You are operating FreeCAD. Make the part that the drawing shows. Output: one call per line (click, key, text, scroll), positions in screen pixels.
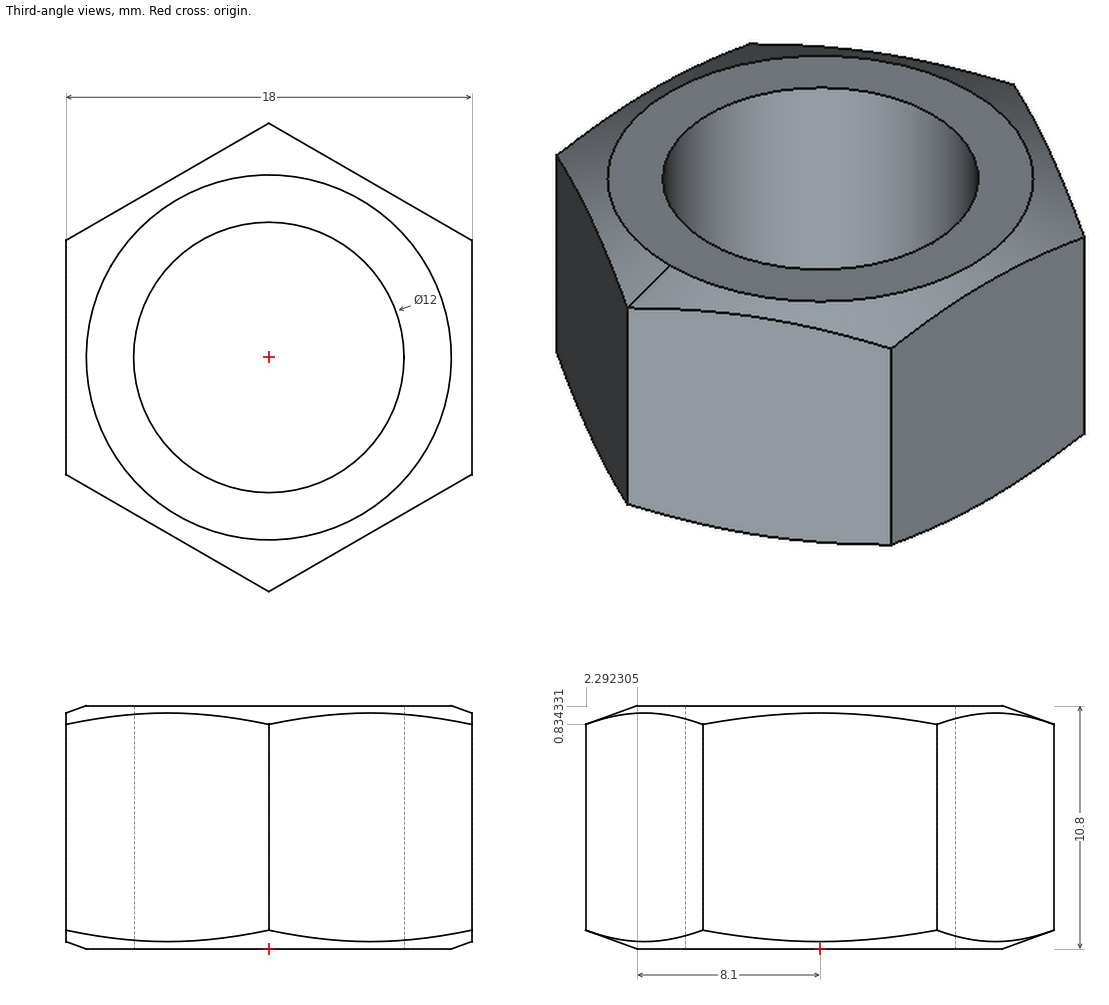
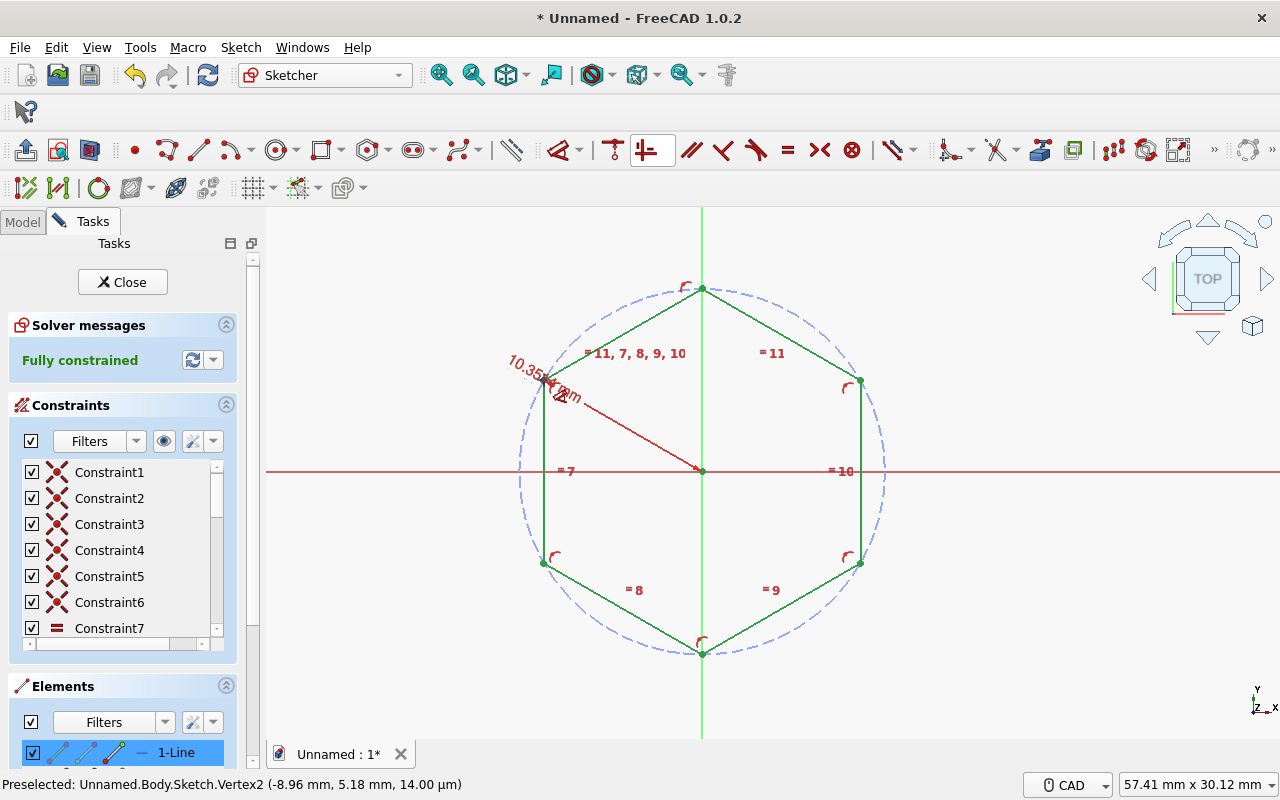
click(861, 563)
click(629, 597)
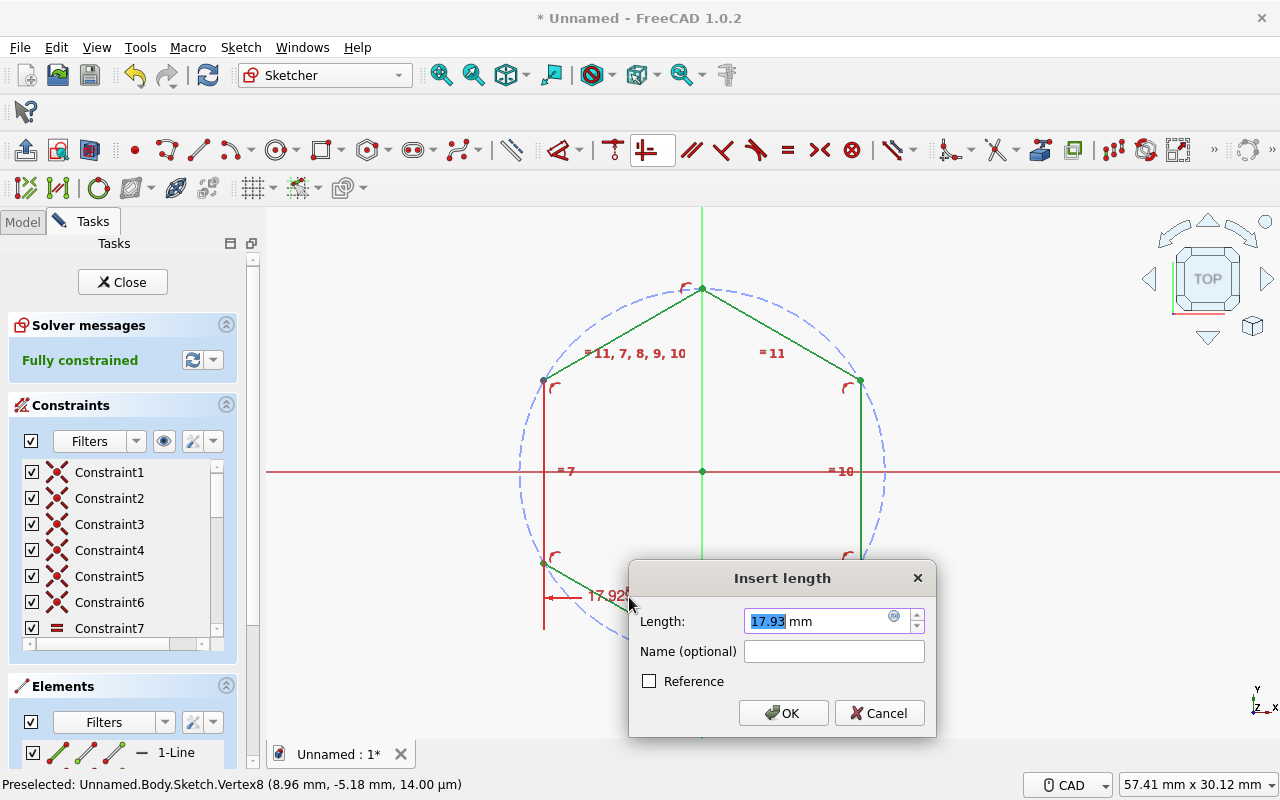
text(18)
key(Return)
key(Escape)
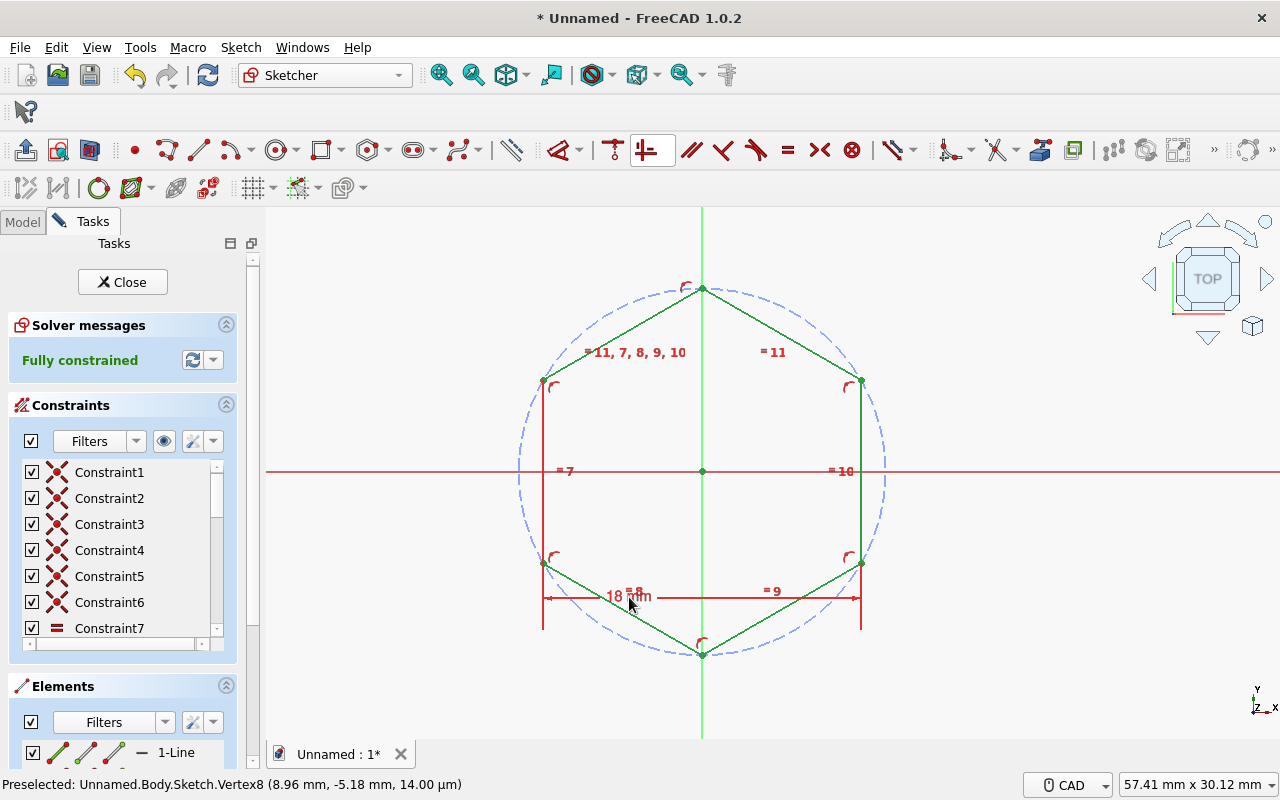
click(123, 282)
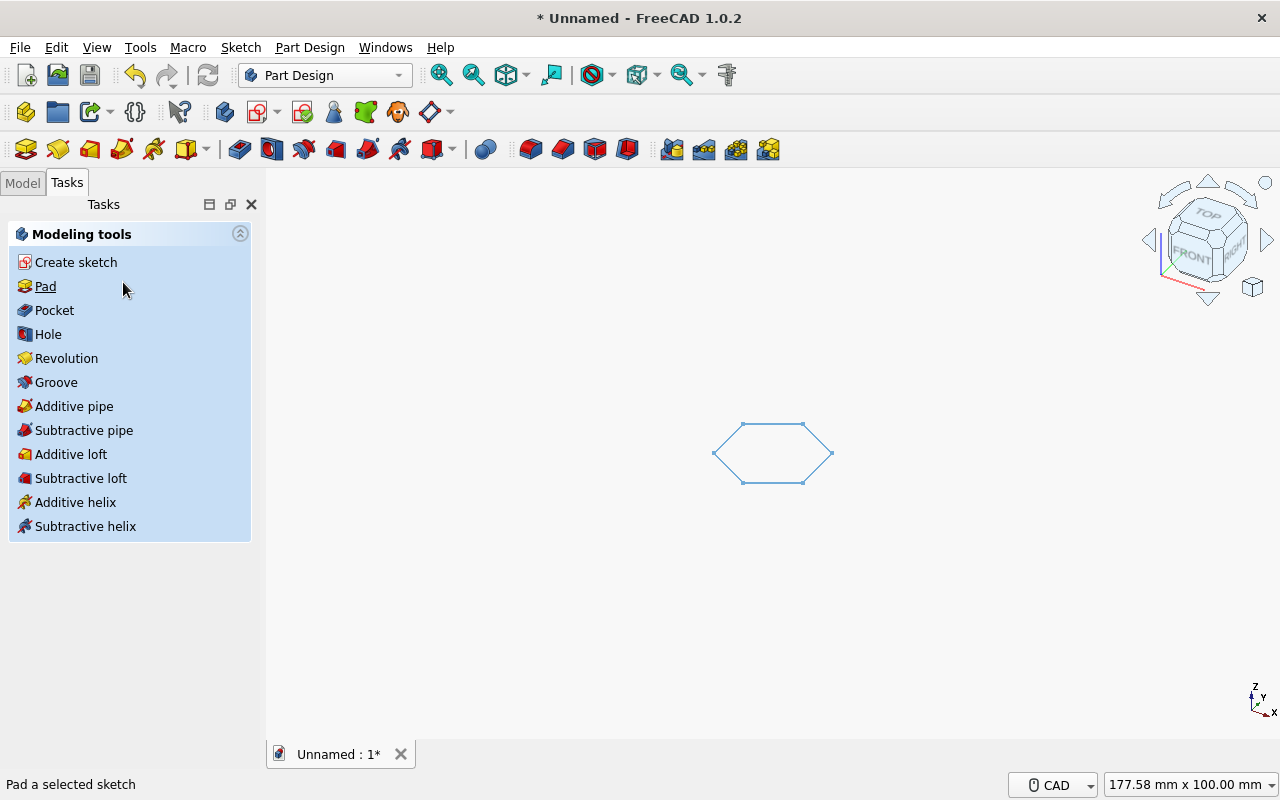
click(26, 150)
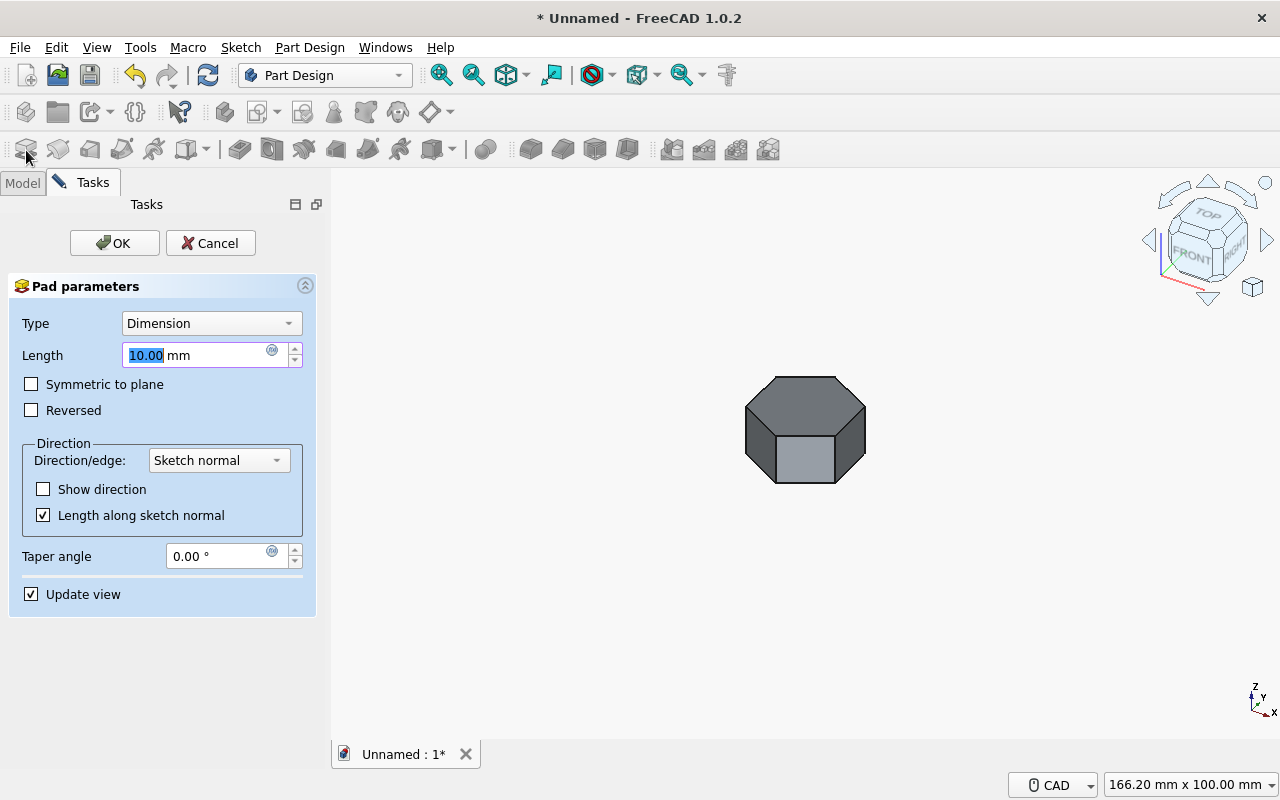
text(10.8)
key(Tab)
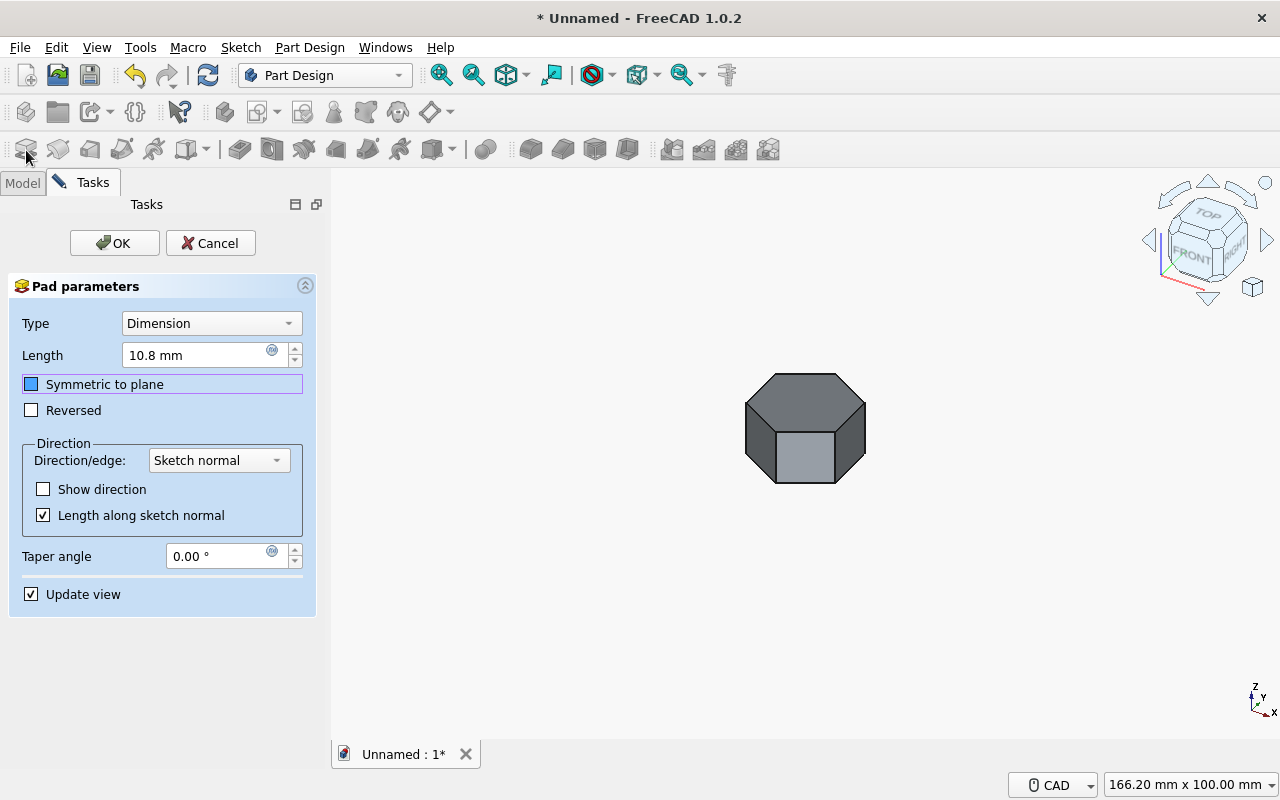
click(115, 243)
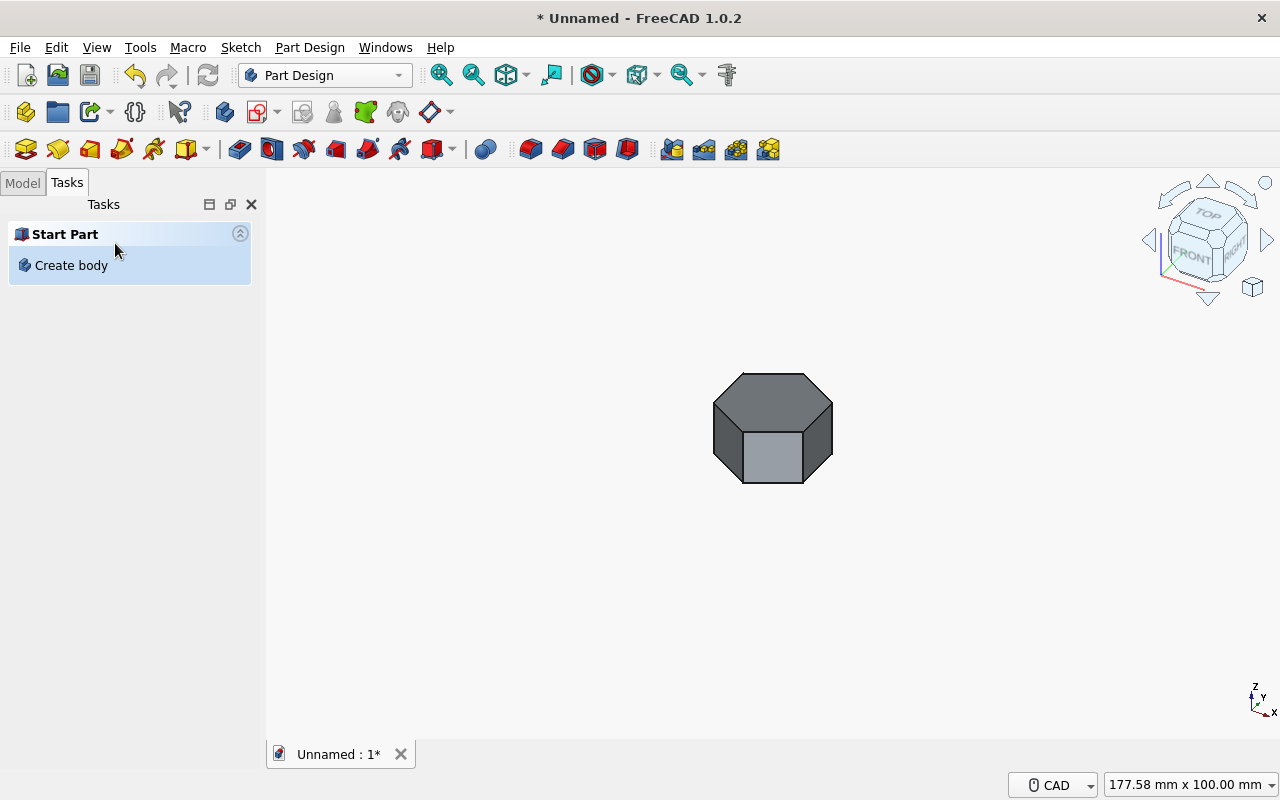
click(442, 76)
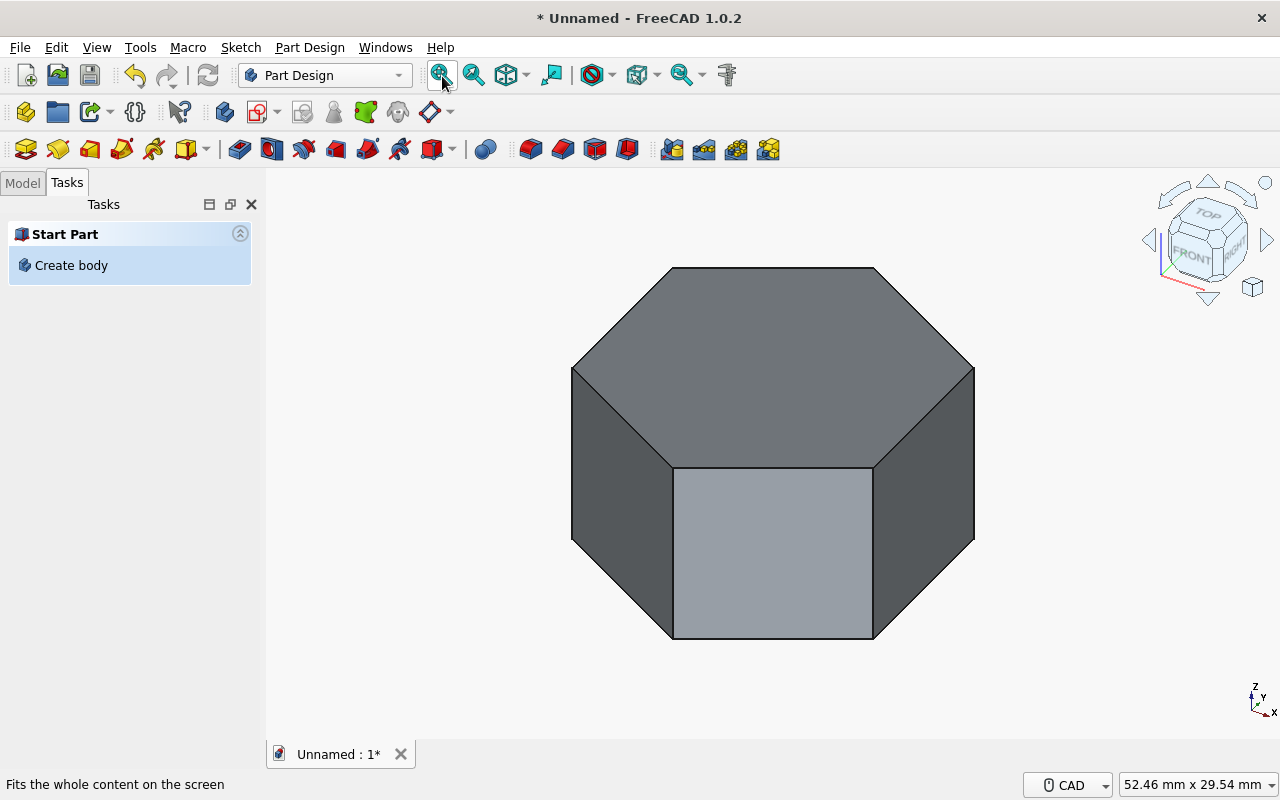
click(258, 112)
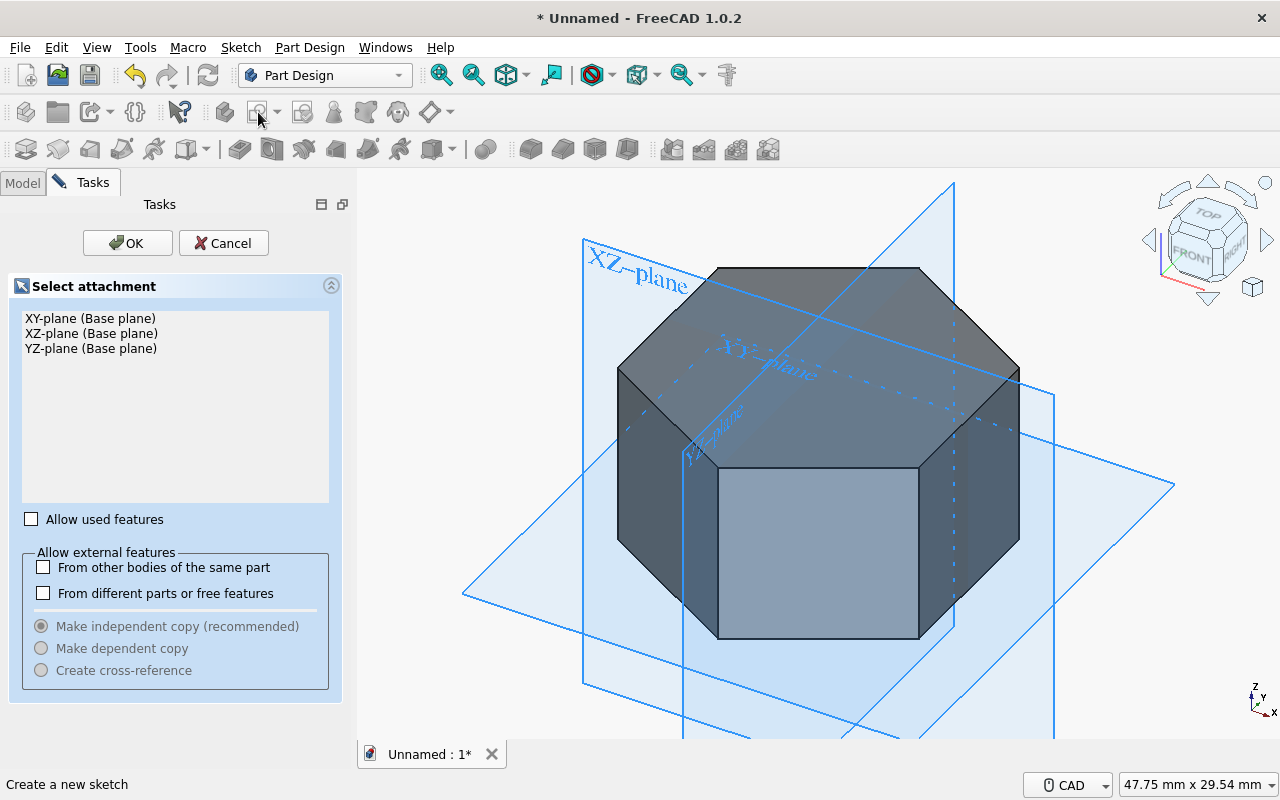
click(82, 348)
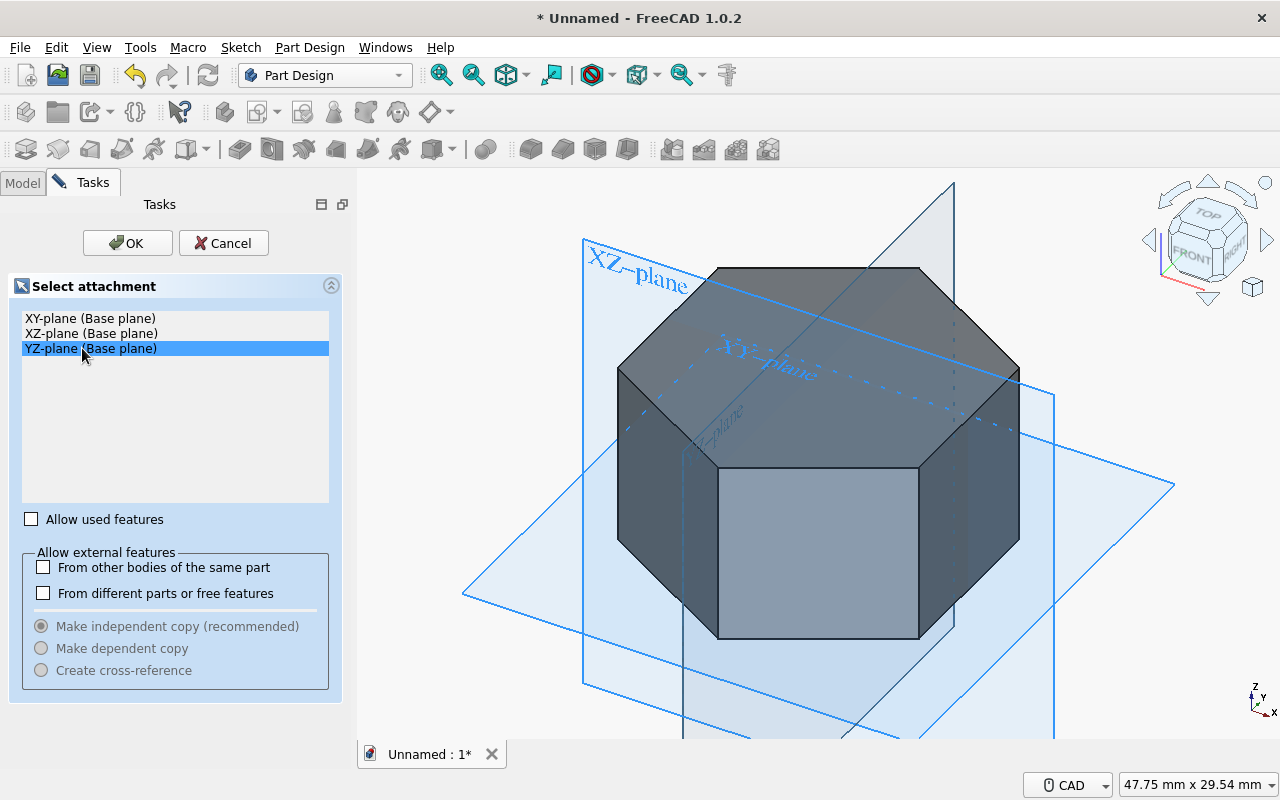
click(128, 243)